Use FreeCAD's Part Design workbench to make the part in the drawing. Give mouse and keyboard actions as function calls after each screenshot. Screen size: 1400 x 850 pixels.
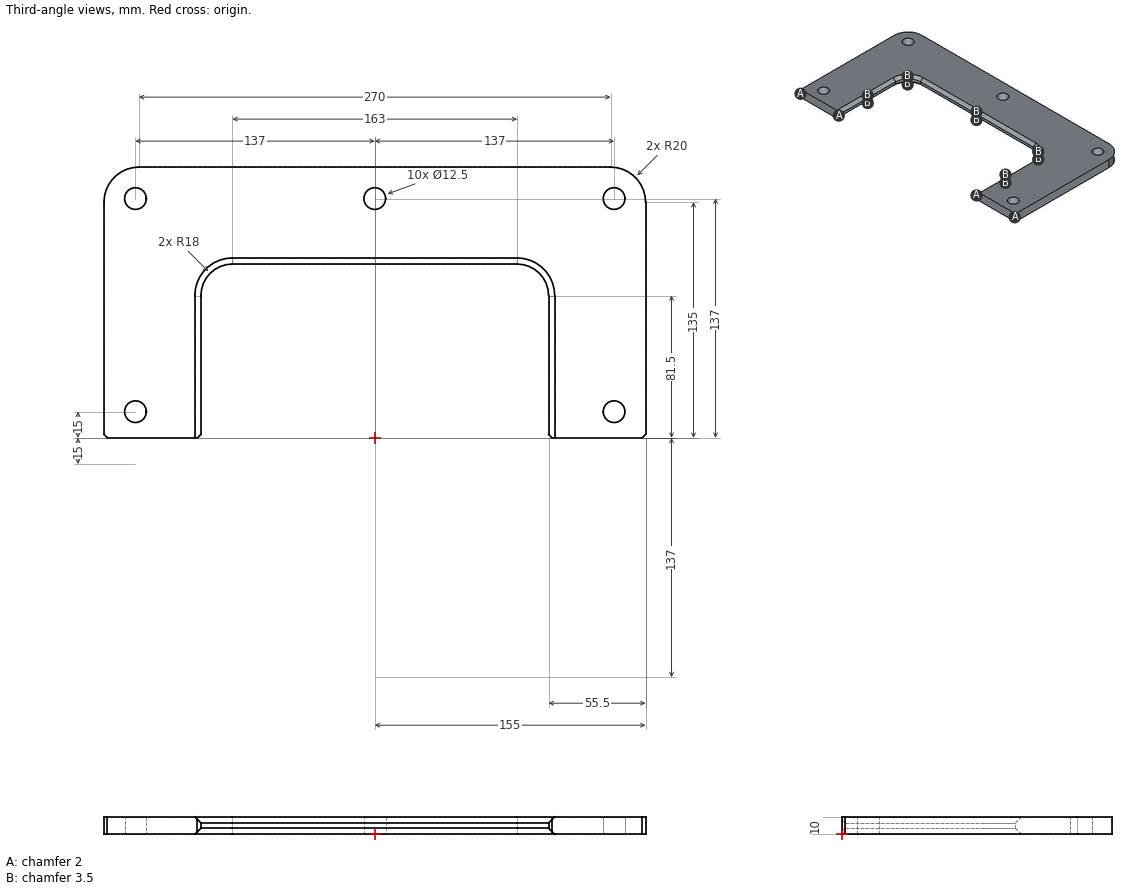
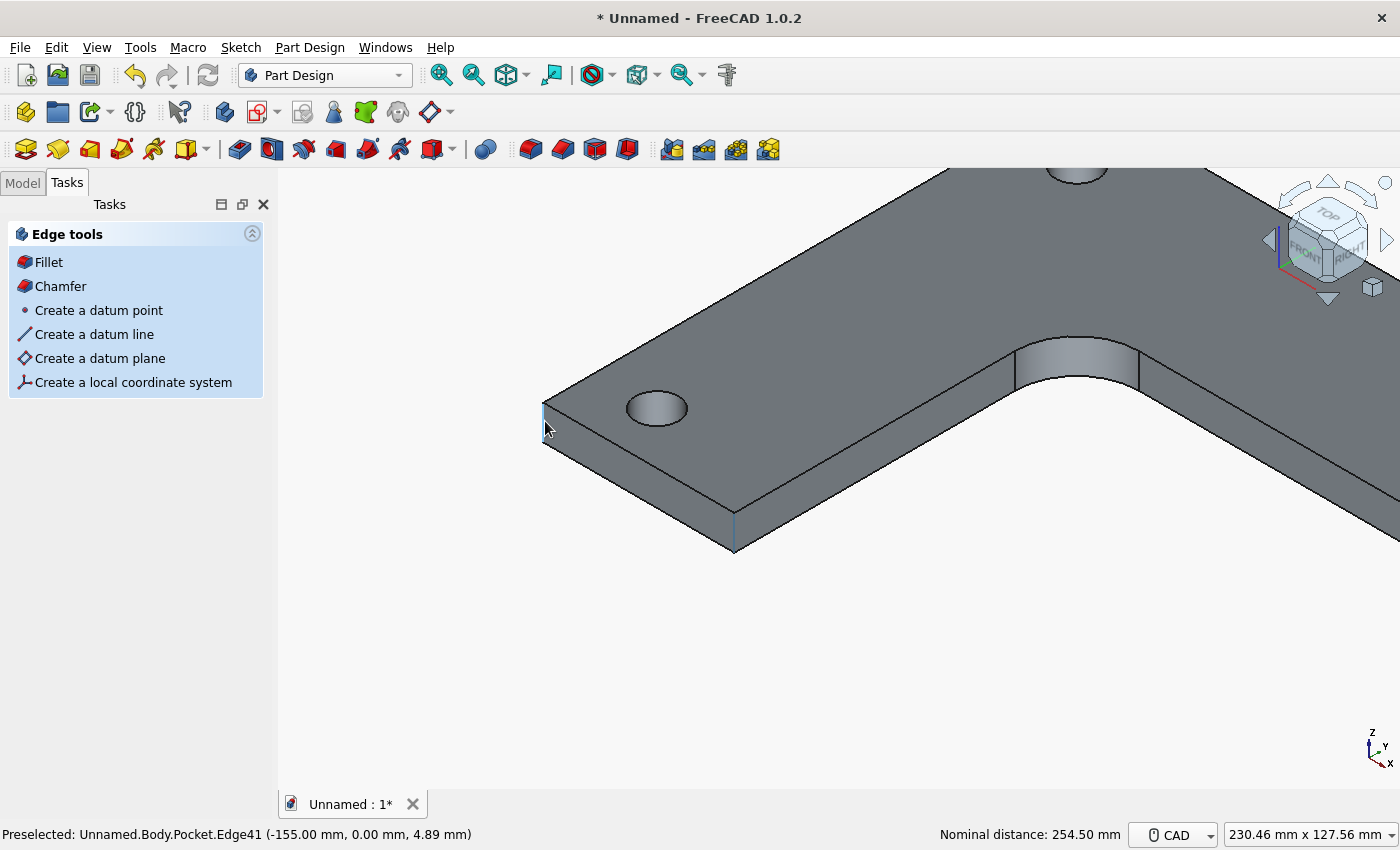
key(v)
key(f)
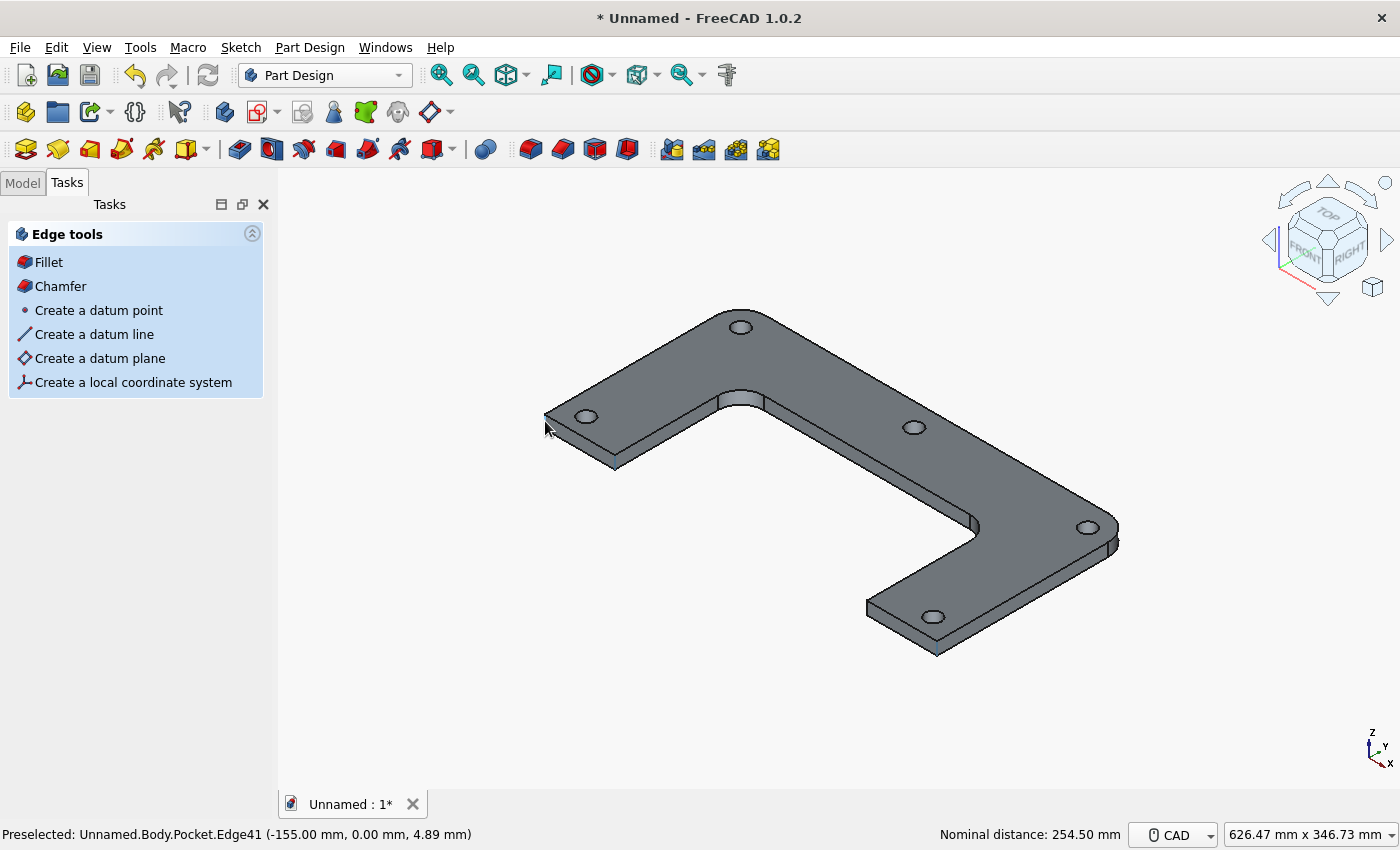
key(2)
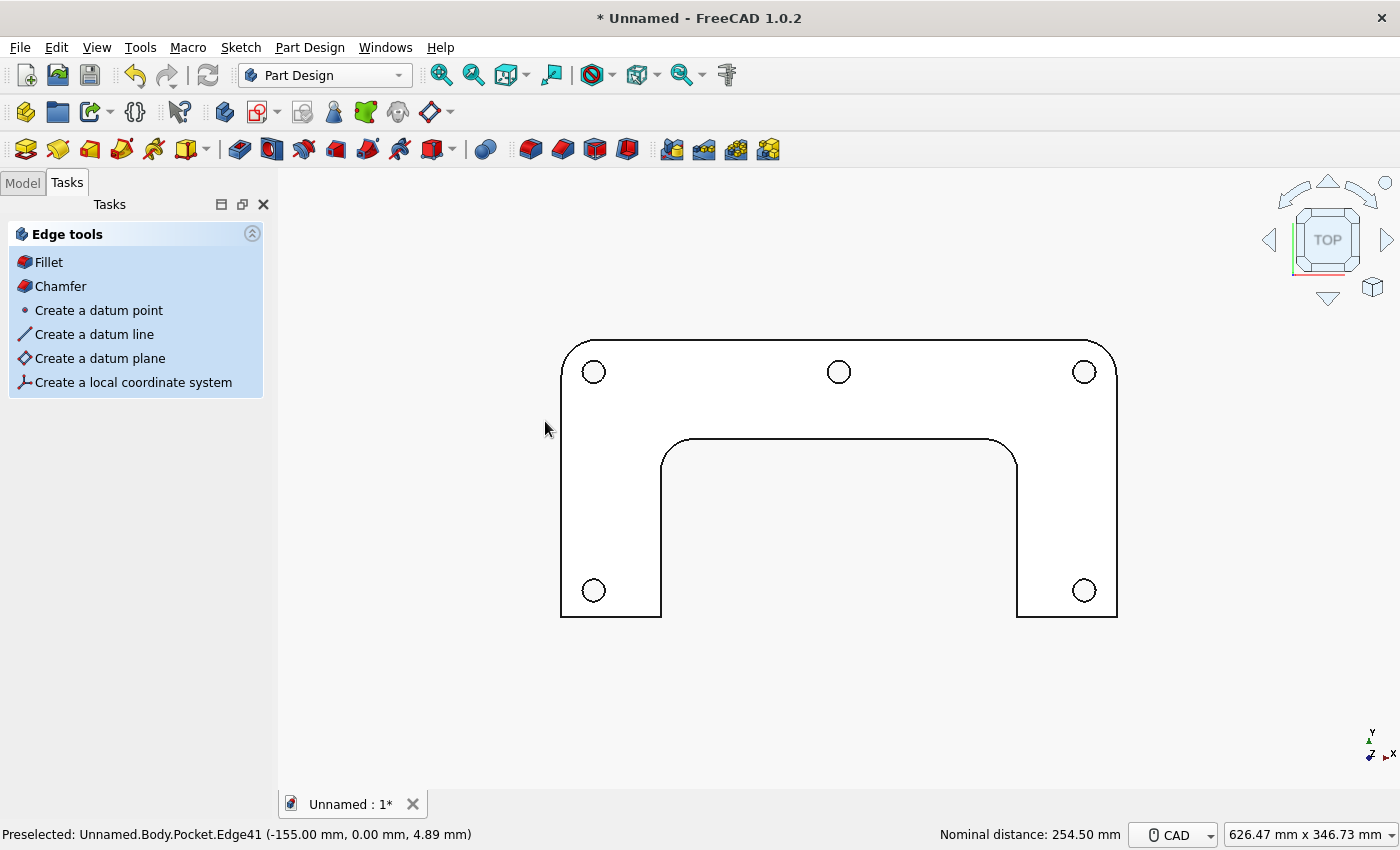
scroll(561, 616, up, 5)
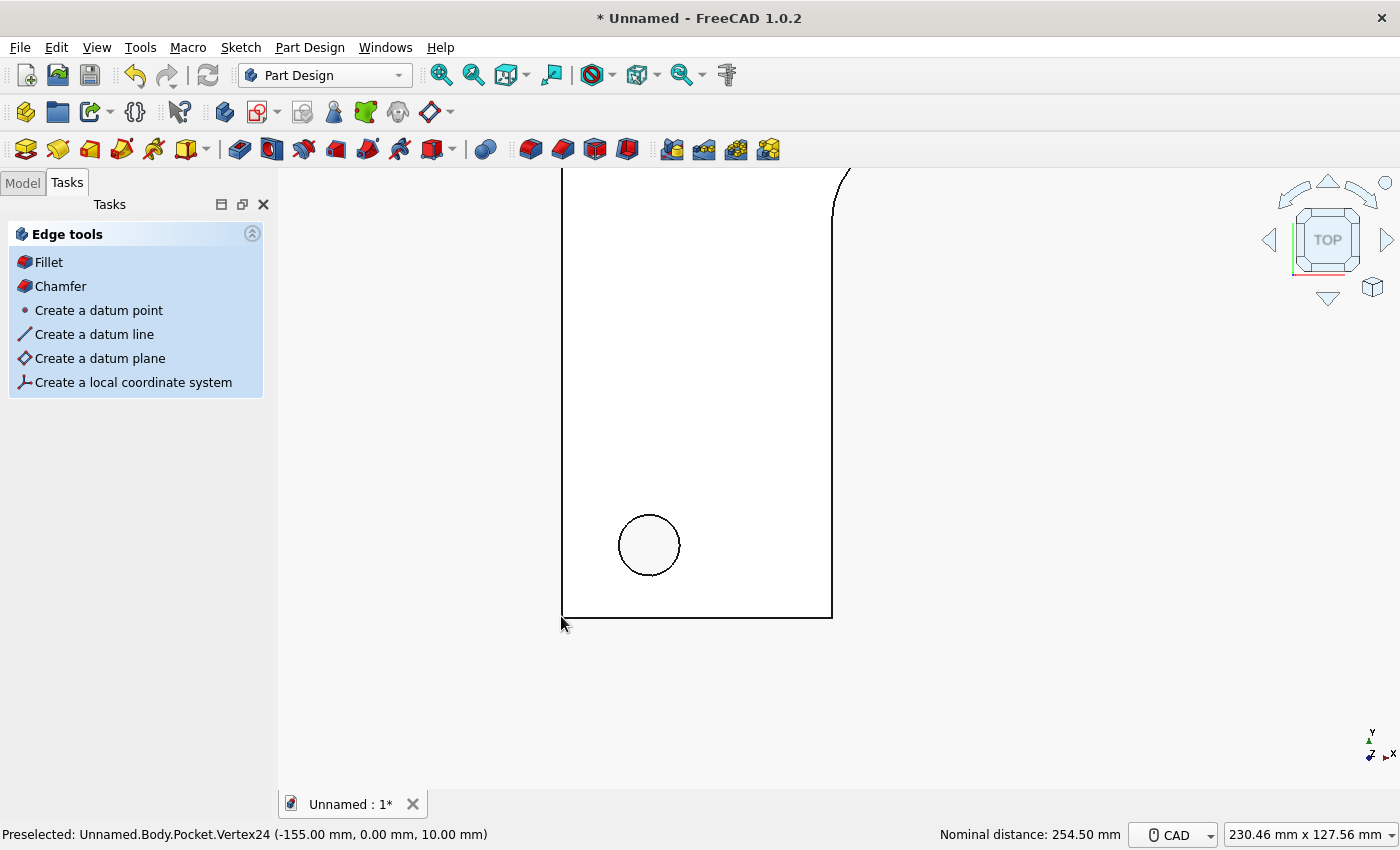
key(v)
key(f)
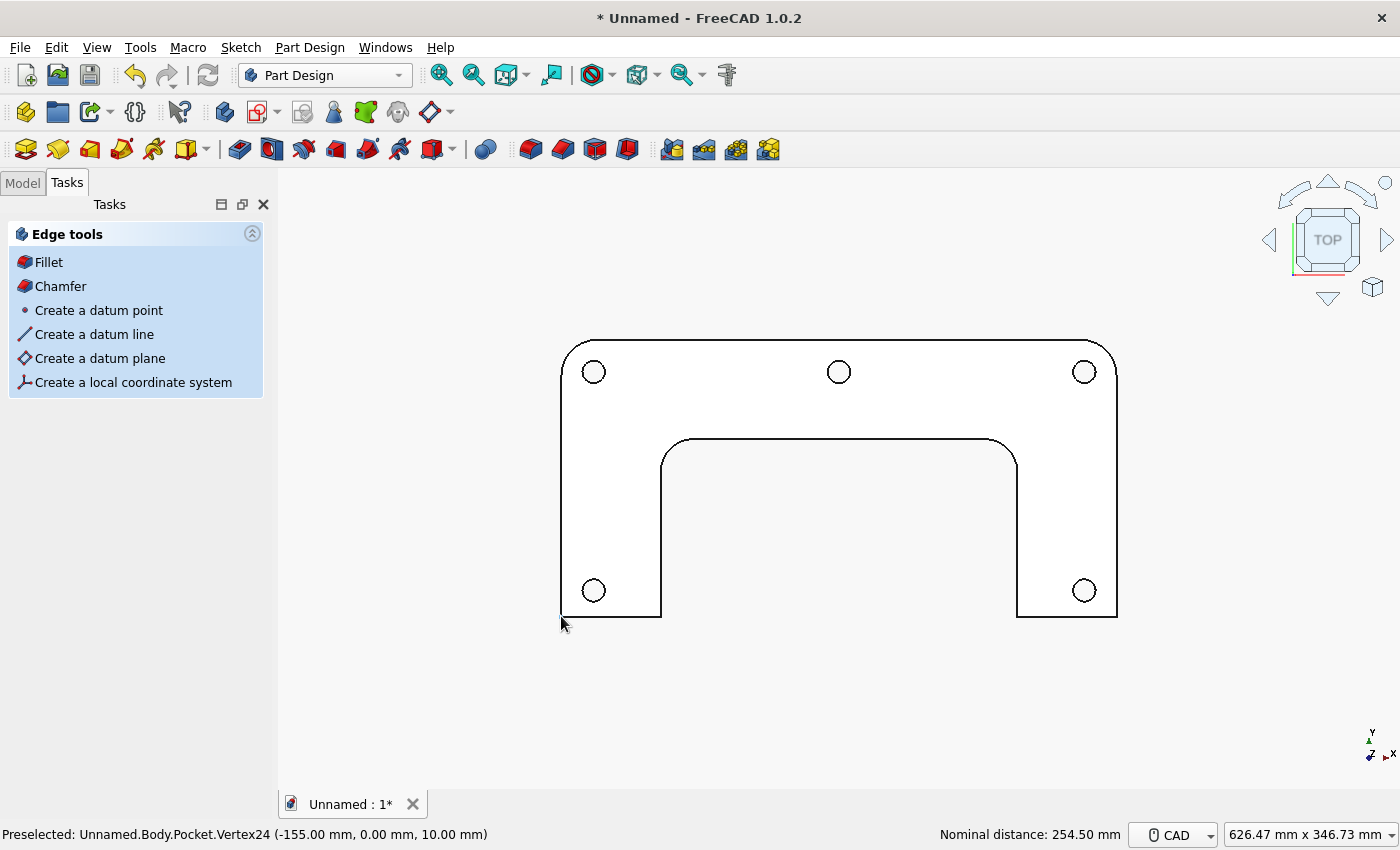
key(1)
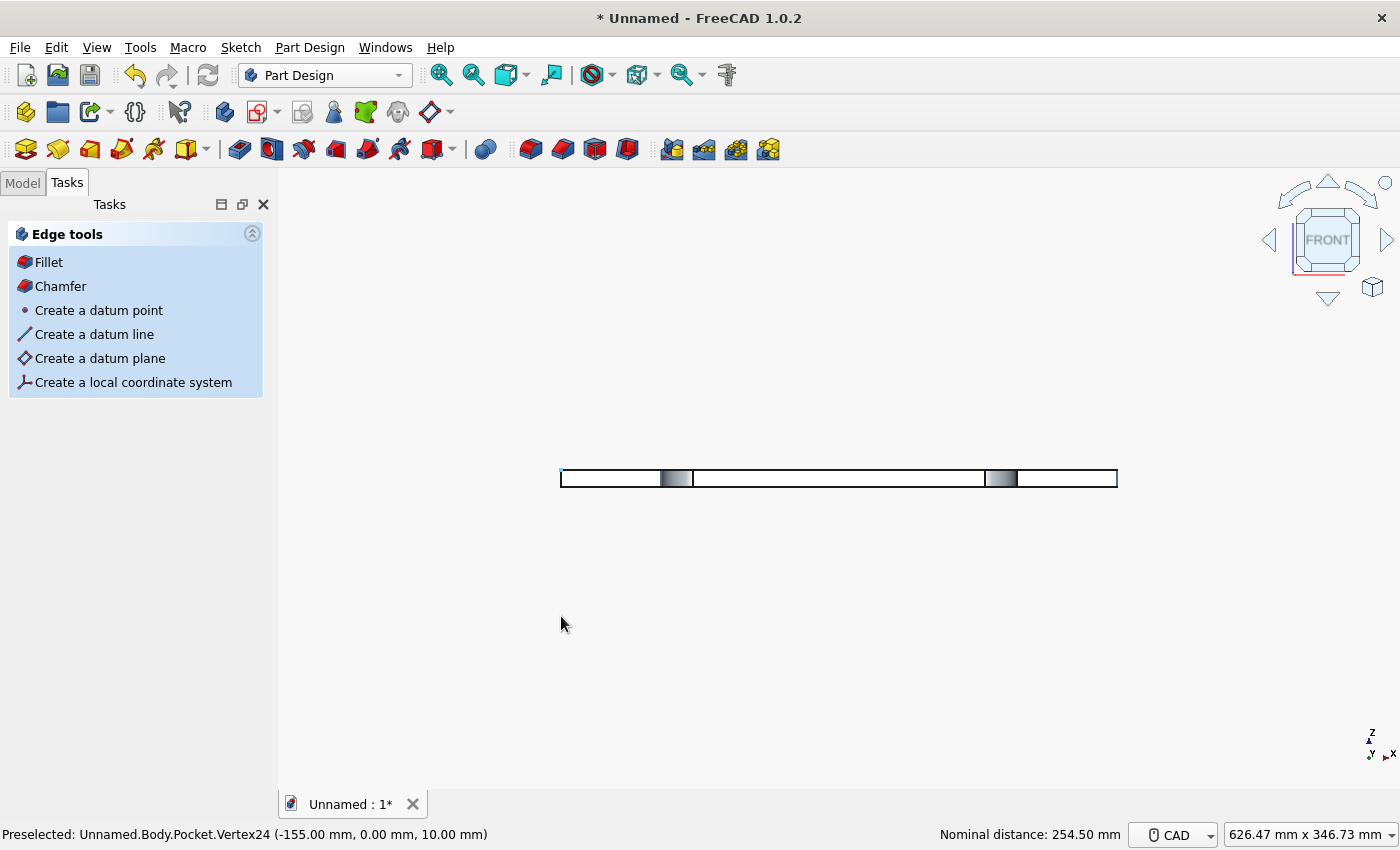
click(561, 478, ctrl)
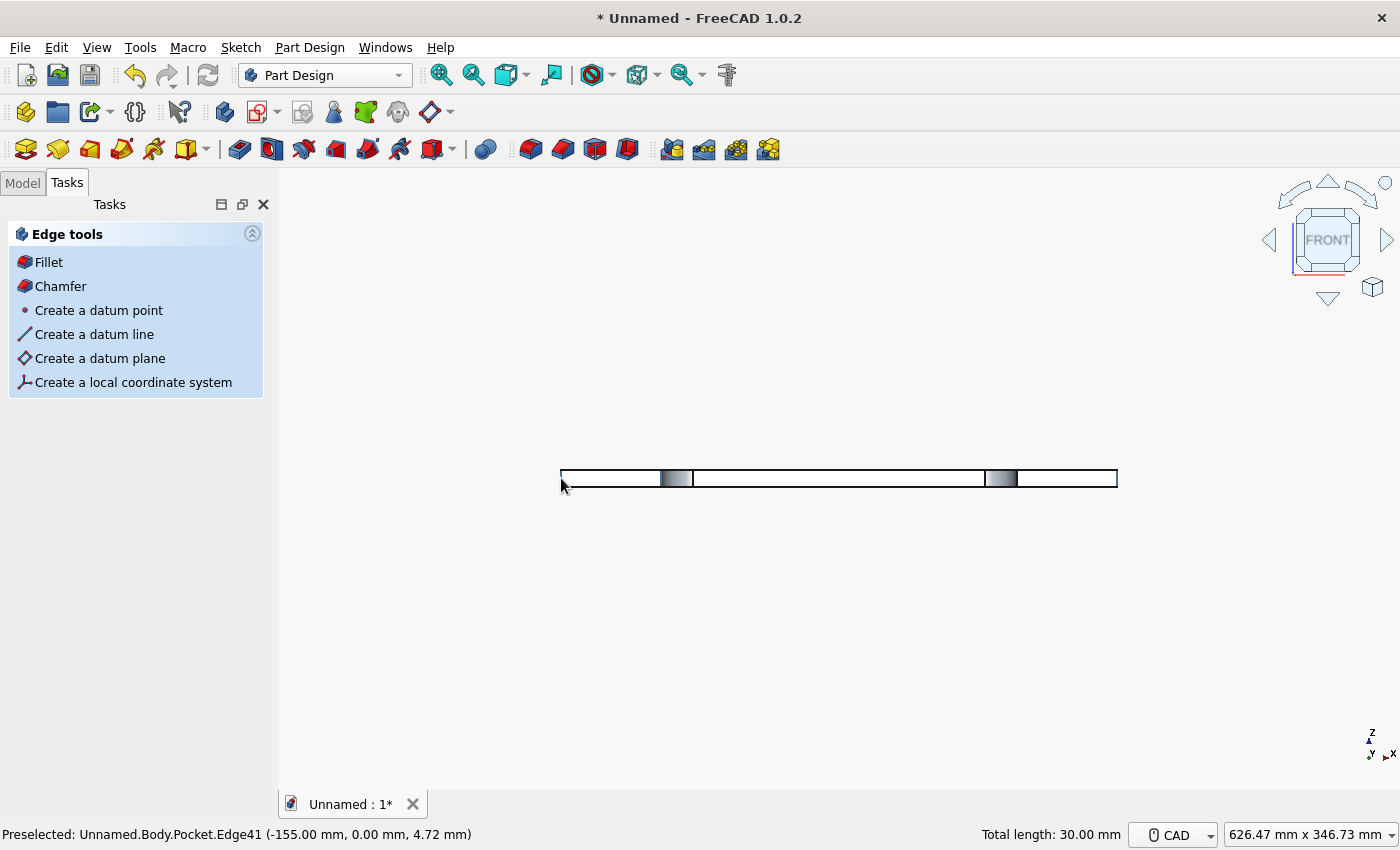
click(1017, 478, ctrl)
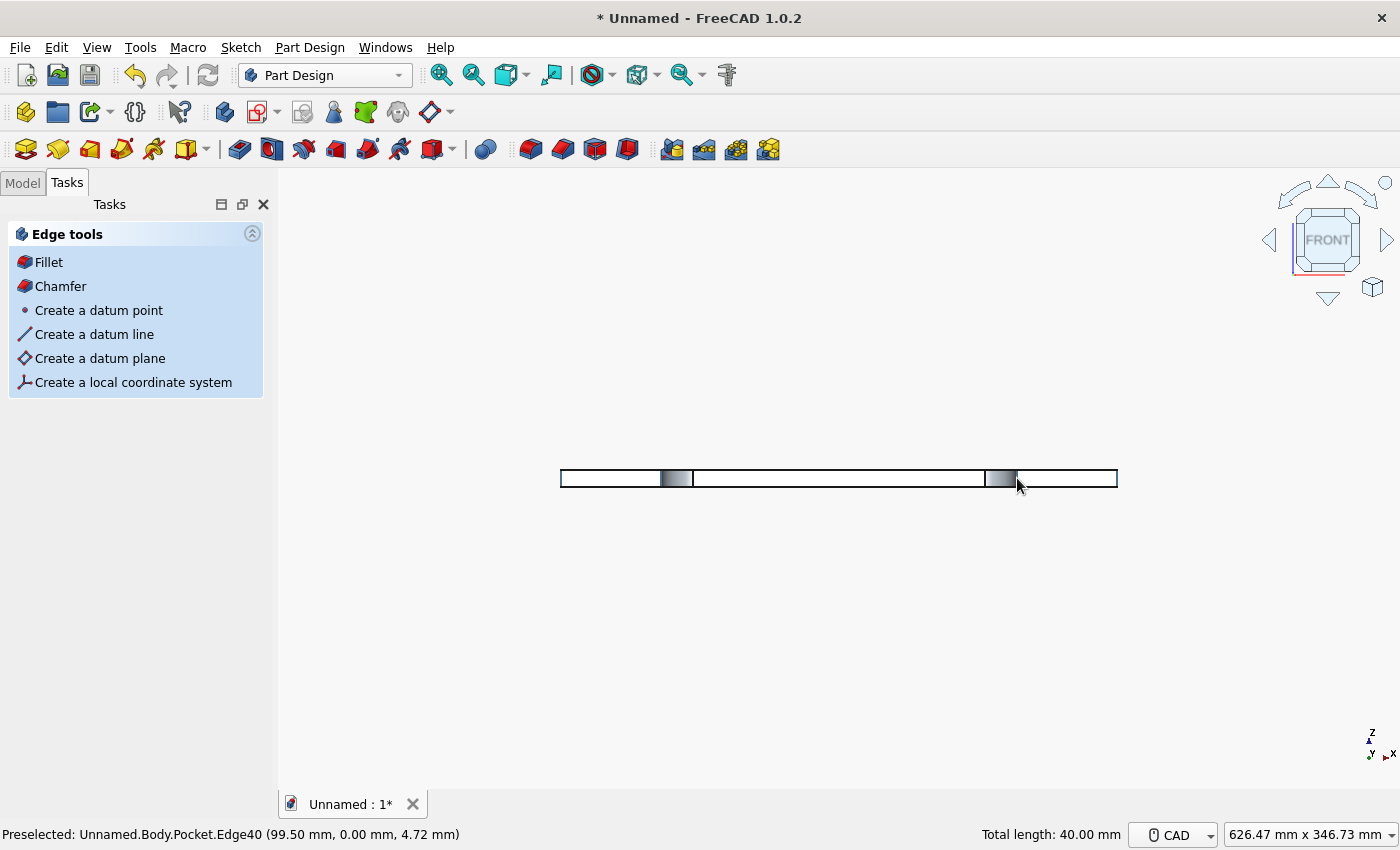
click(564, 150)